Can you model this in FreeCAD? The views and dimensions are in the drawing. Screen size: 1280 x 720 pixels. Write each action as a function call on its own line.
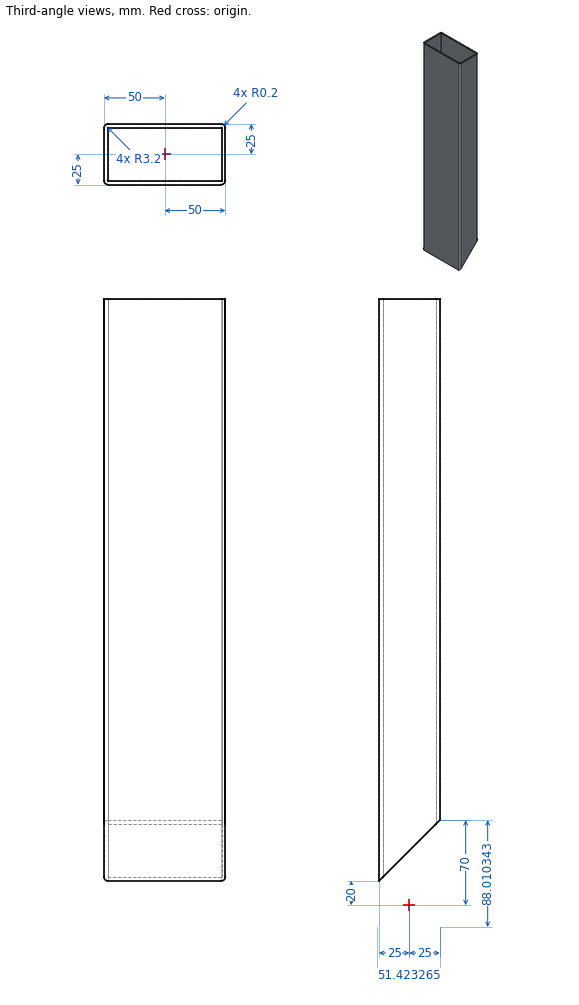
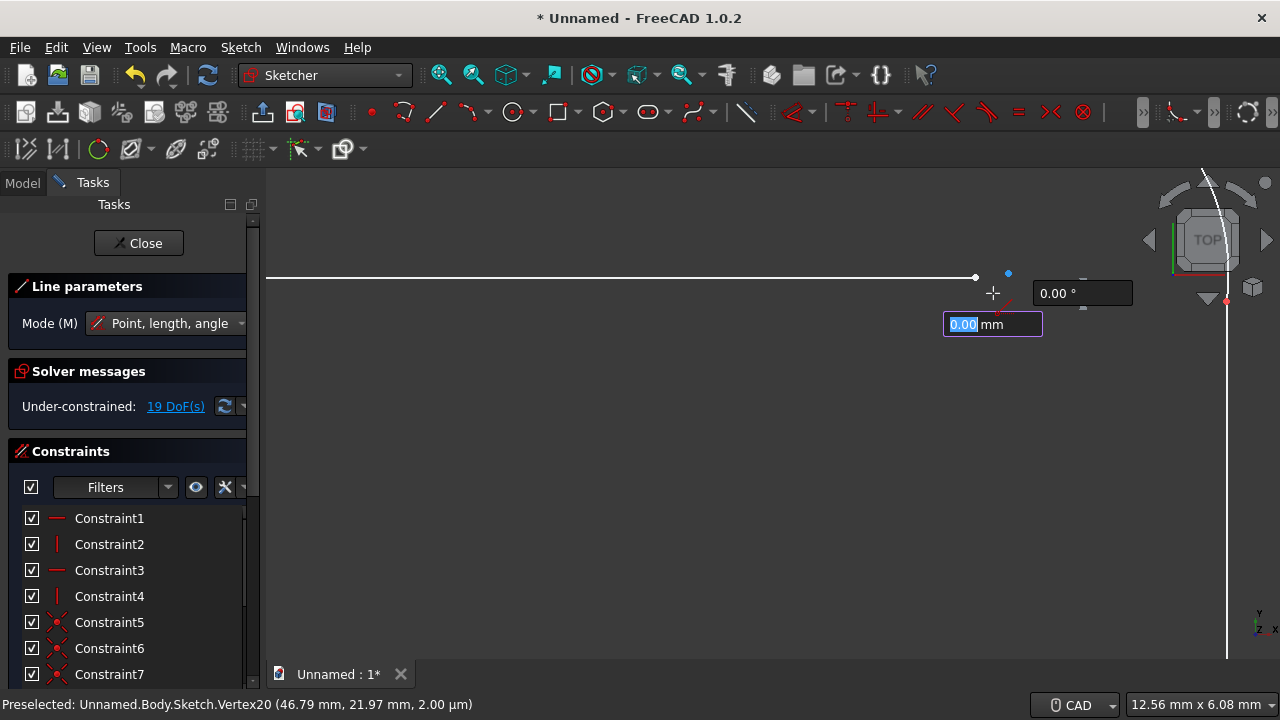
scroll(986, 282, down, 13)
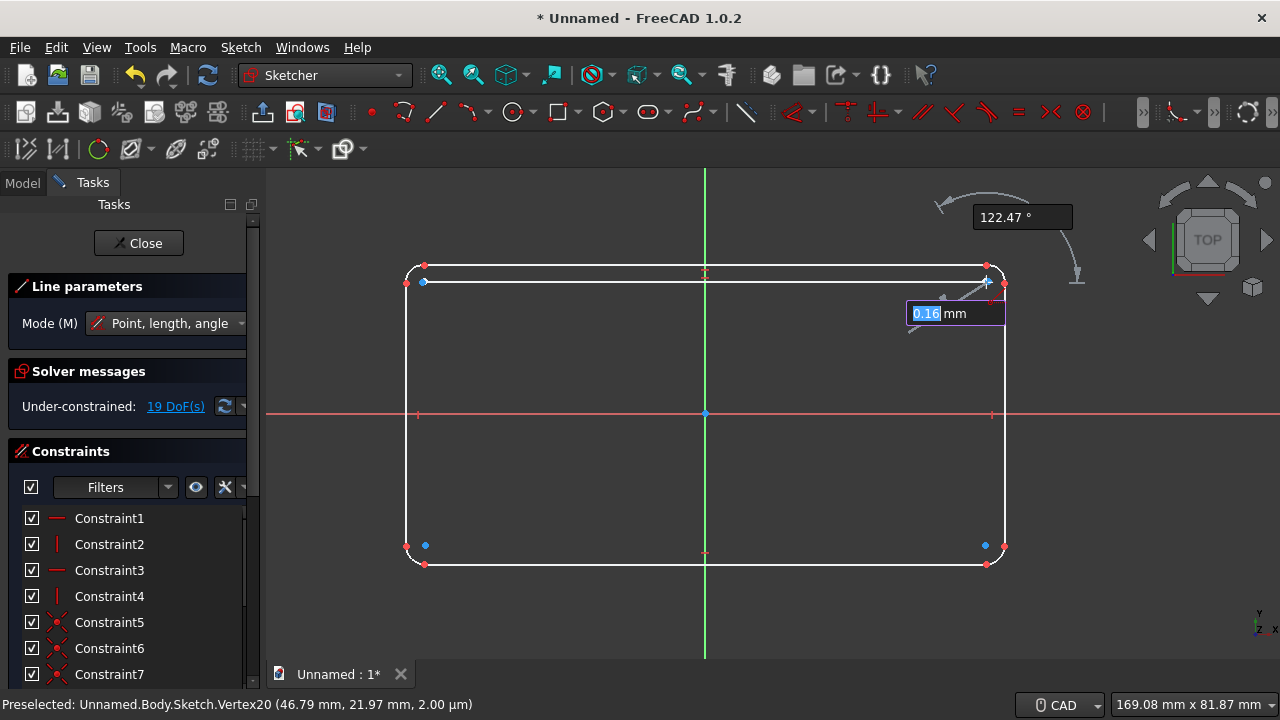
scroll(987, 545, up, 13)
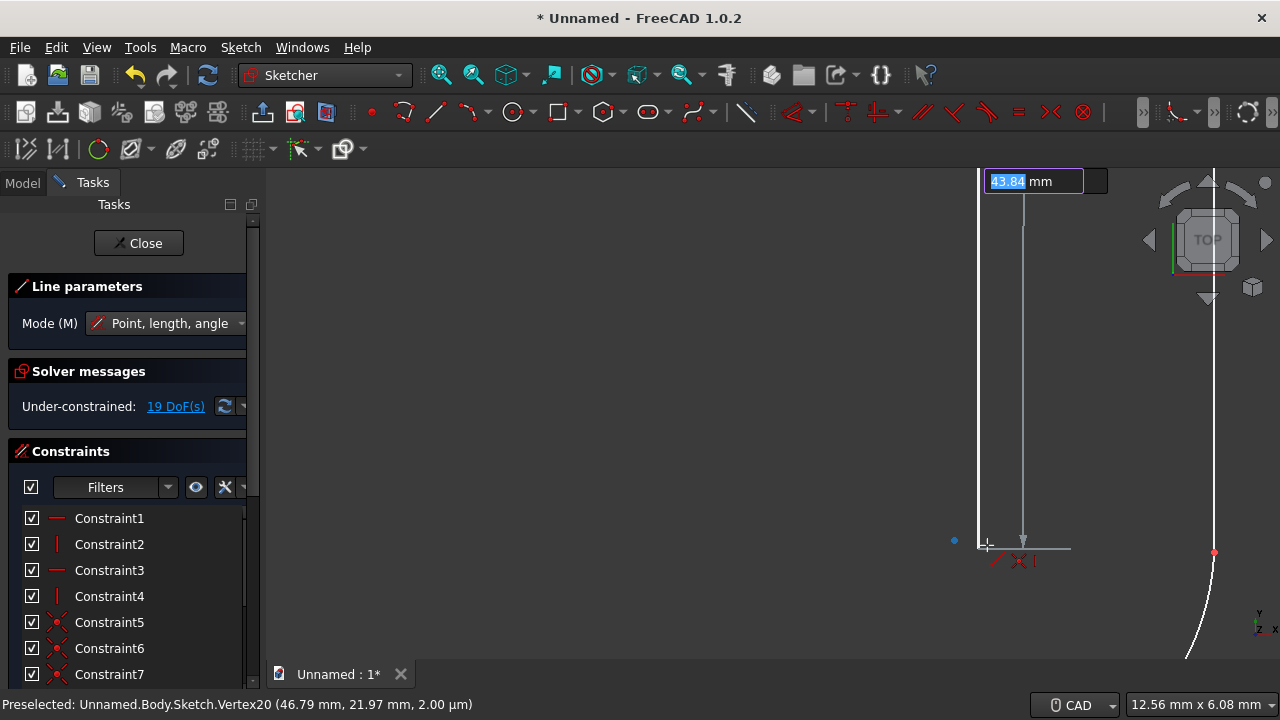
click(981, 529)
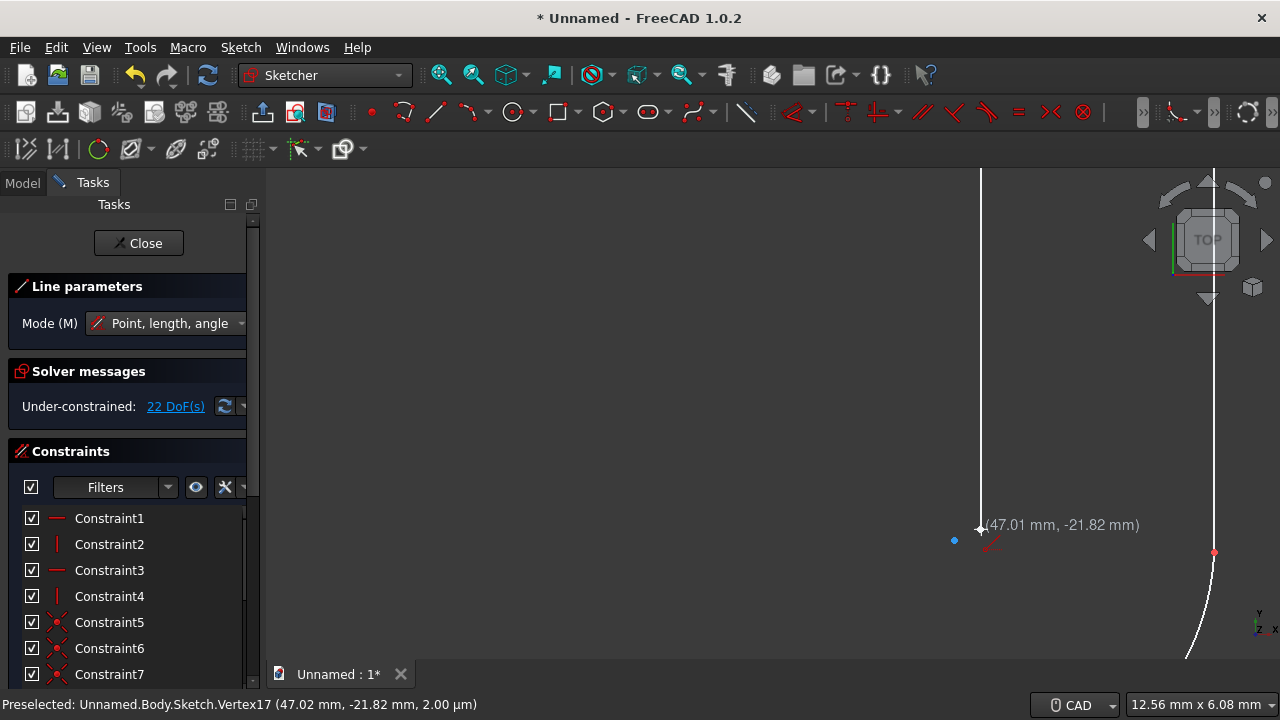
click(964, 545)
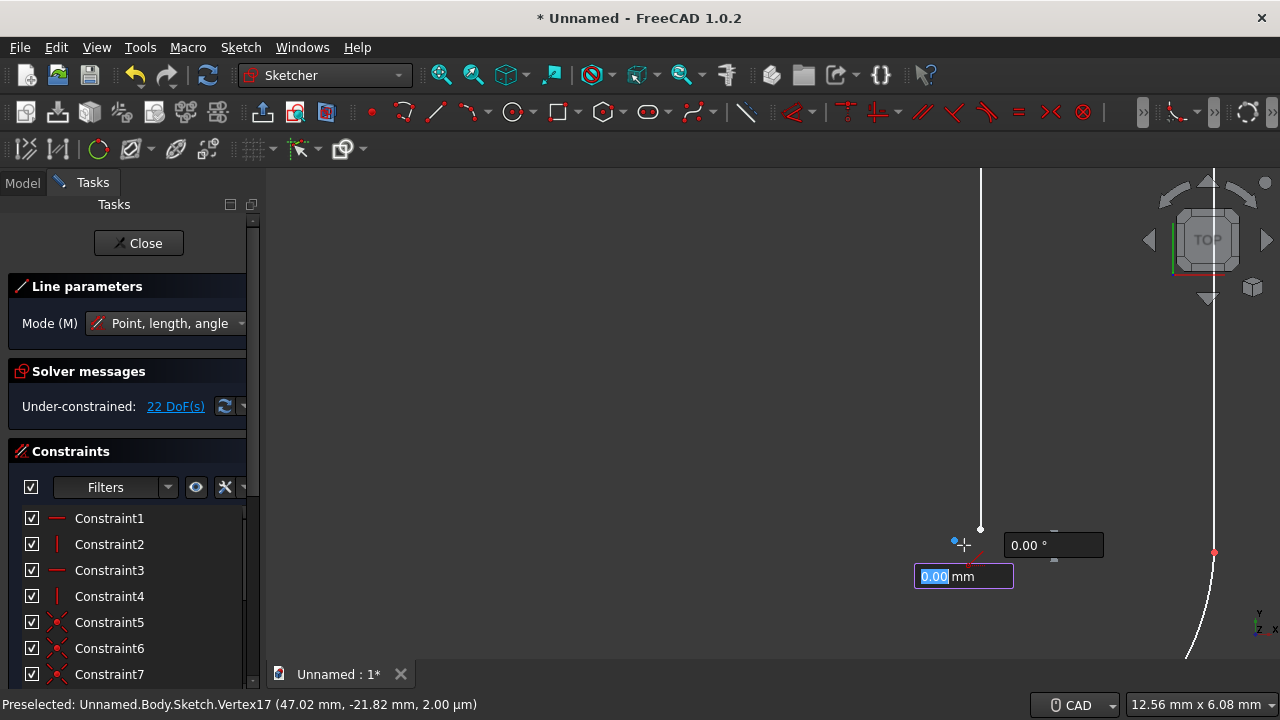
scroll(987, 545, down, 13)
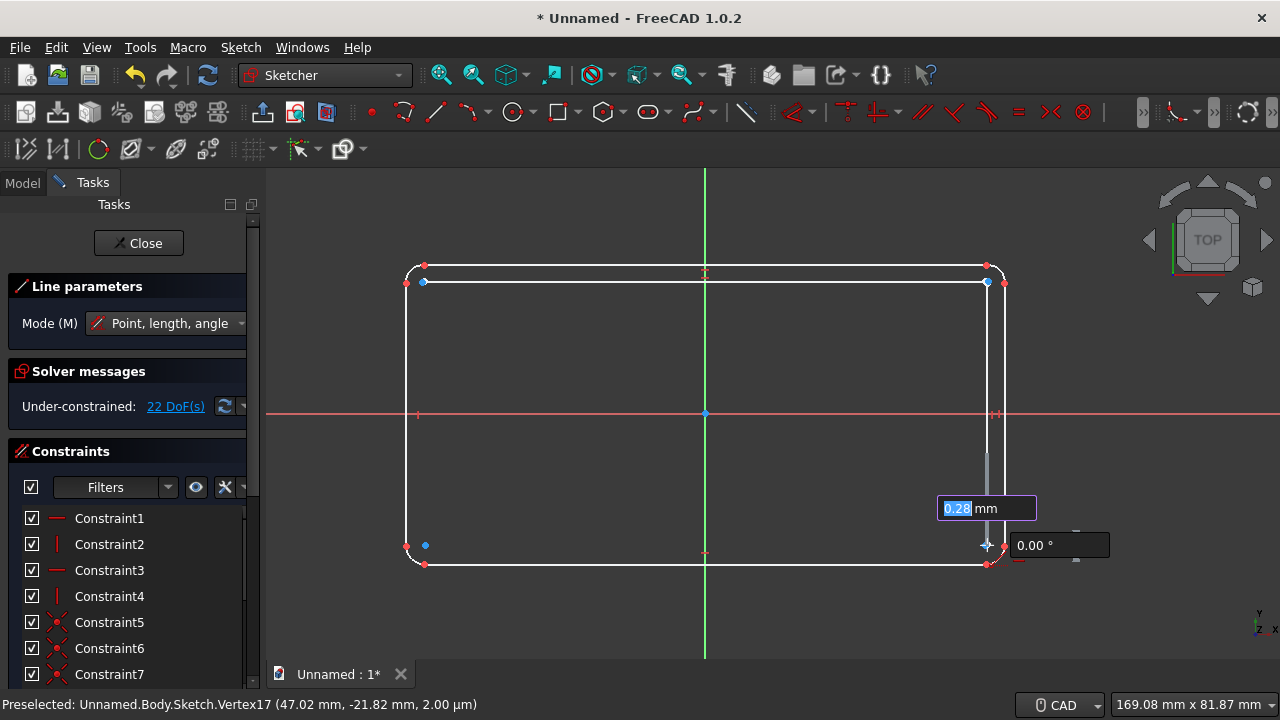
scroll(425, 546, up, 13)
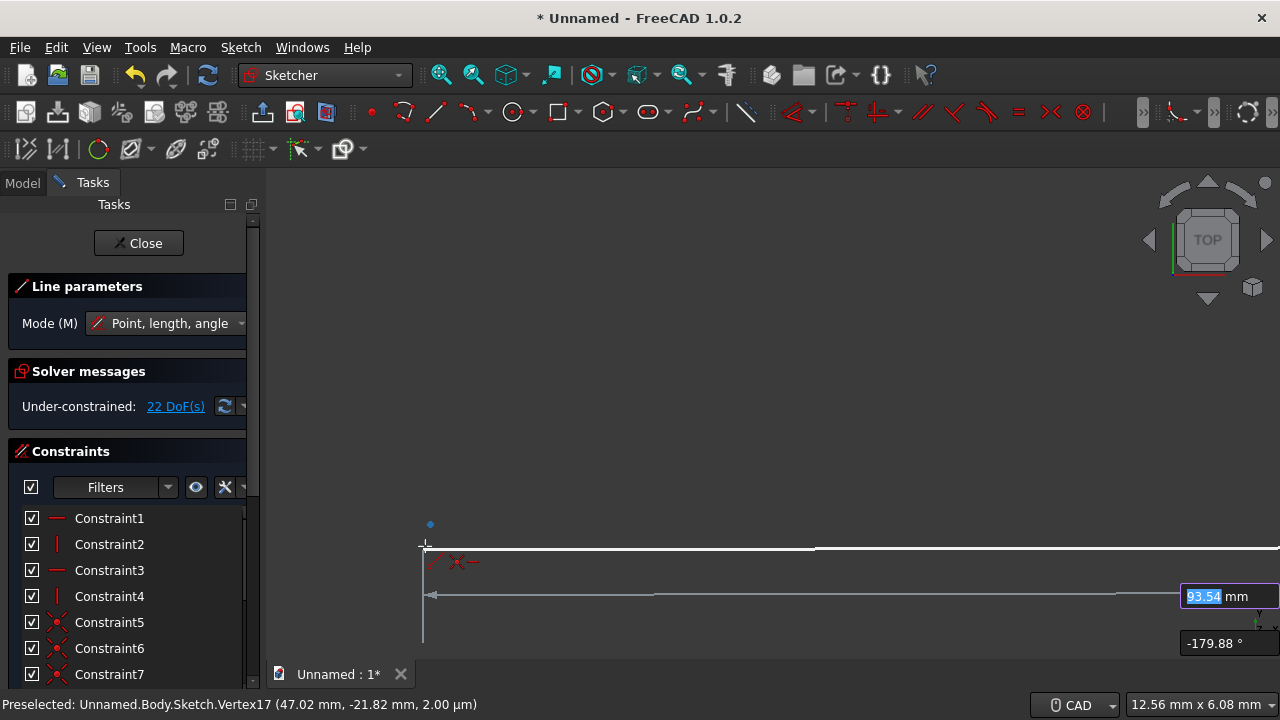
click(418, 533)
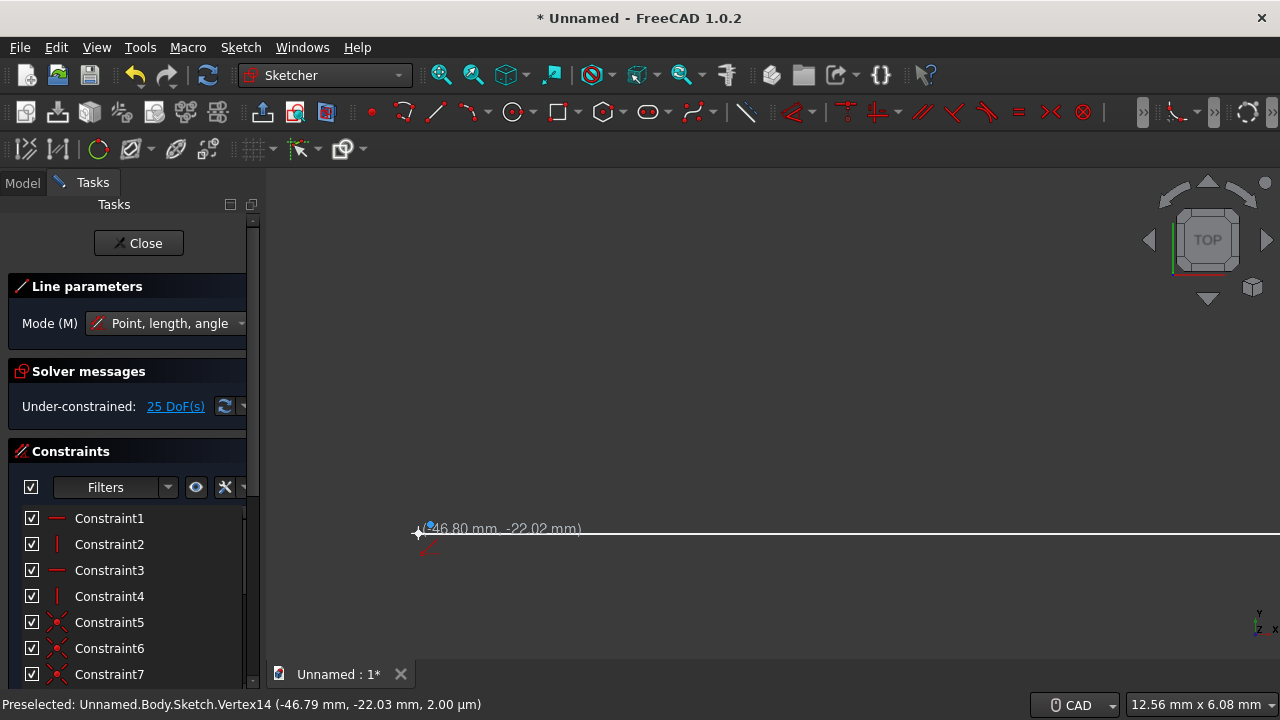
click(402, 516)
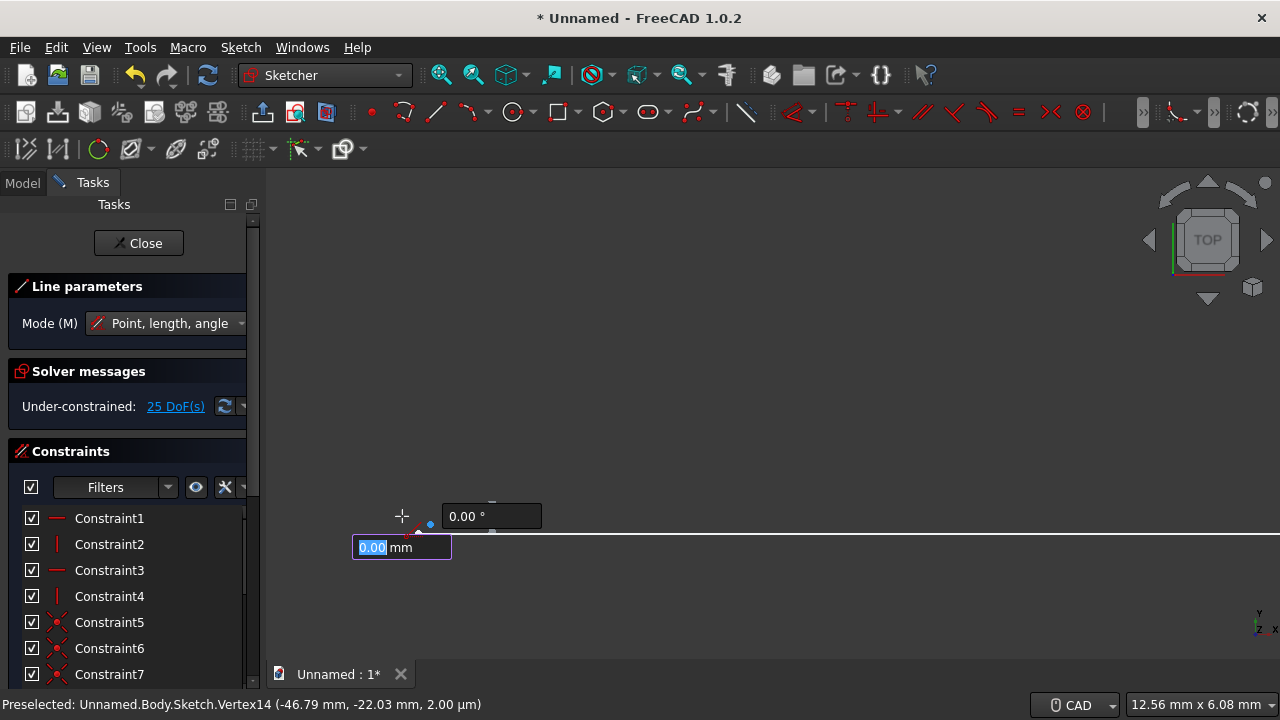
scroll(424, 546, down, 13)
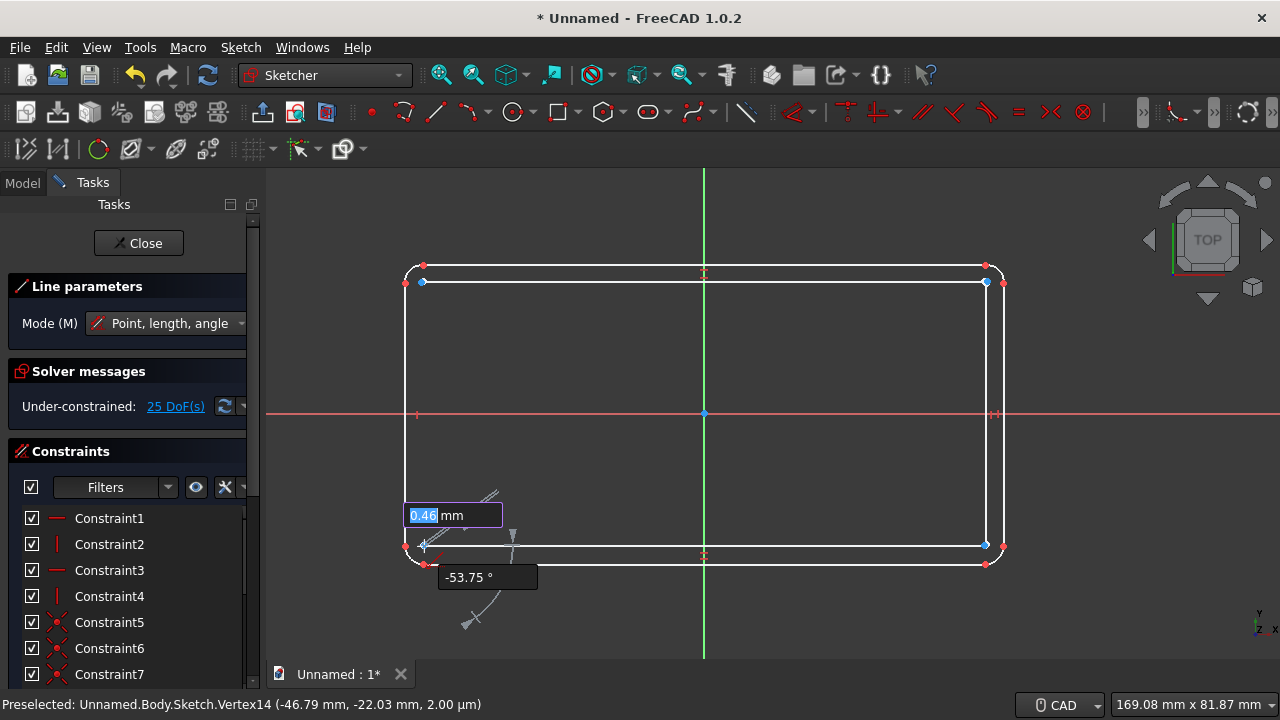
scroll(422, 283, up, 13)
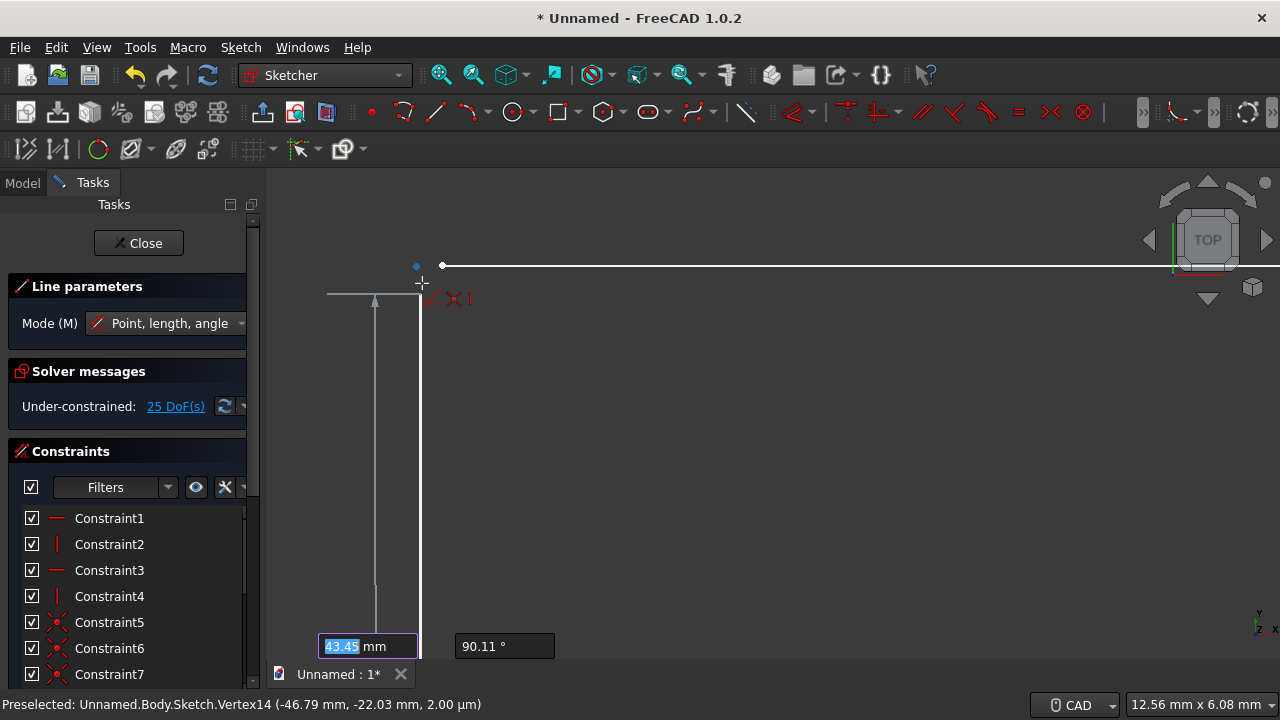
click(427, 281)